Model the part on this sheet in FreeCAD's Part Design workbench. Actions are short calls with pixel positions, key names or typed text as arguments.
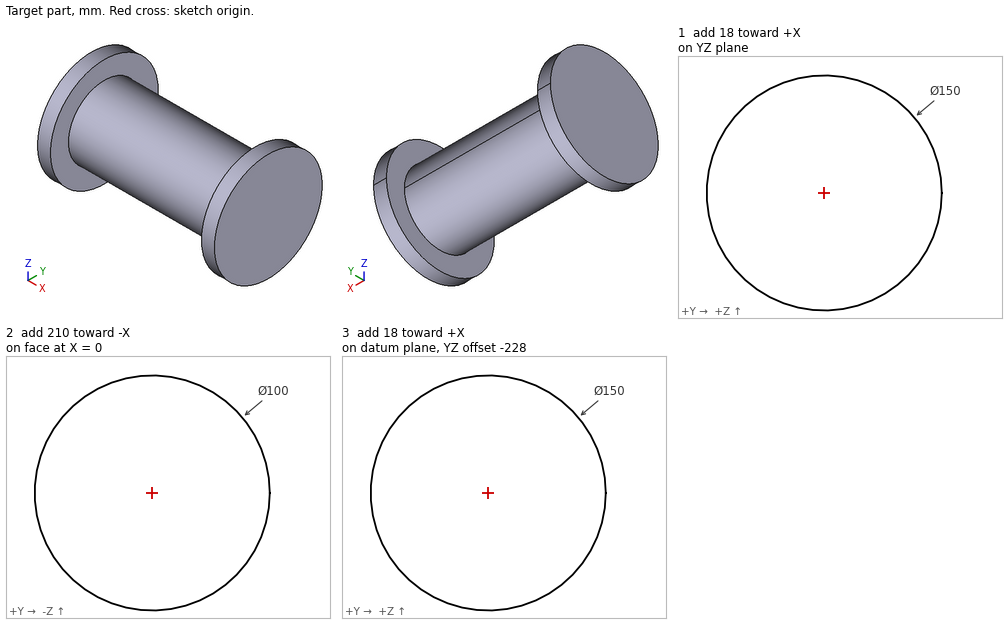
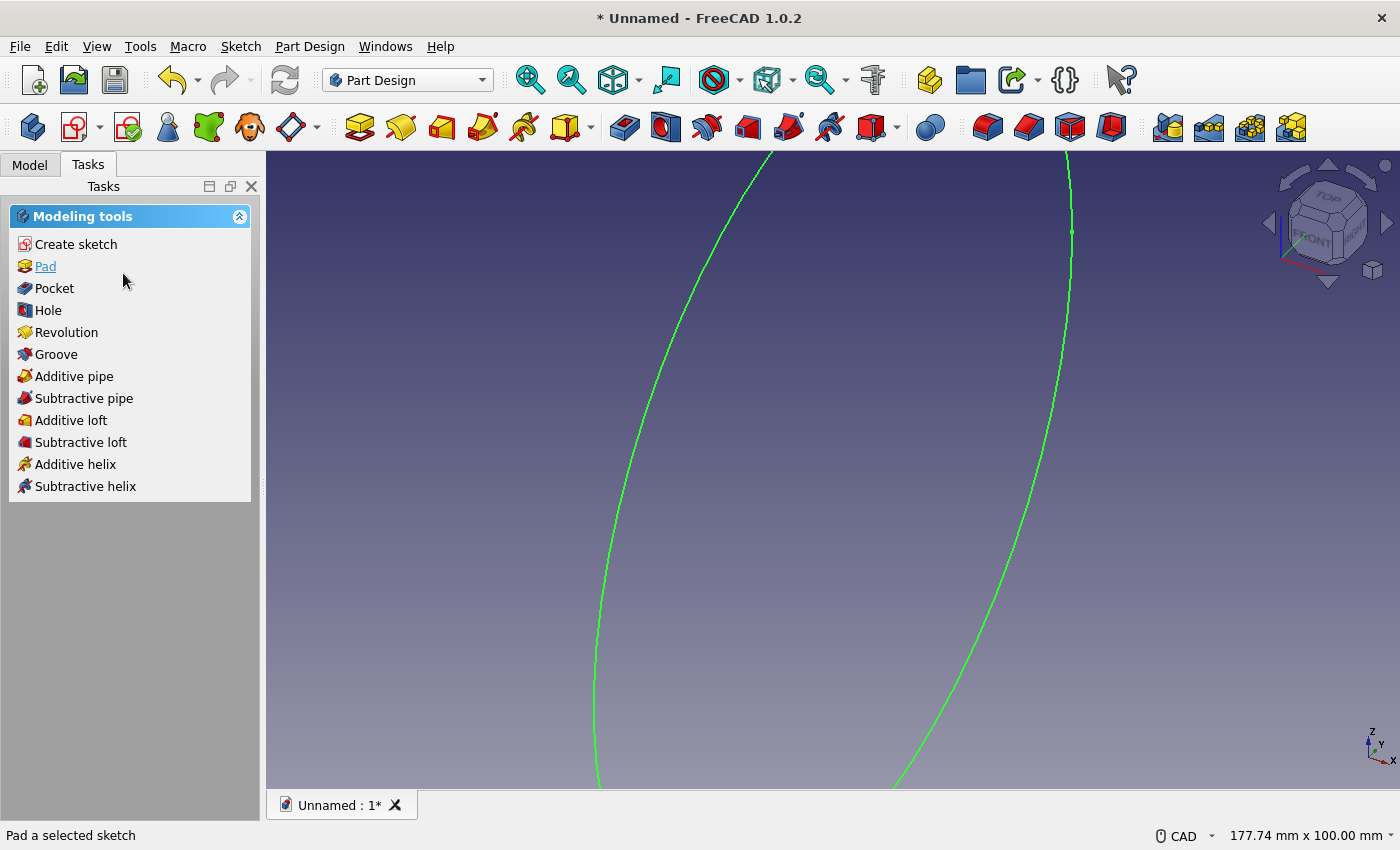
click(360, 128)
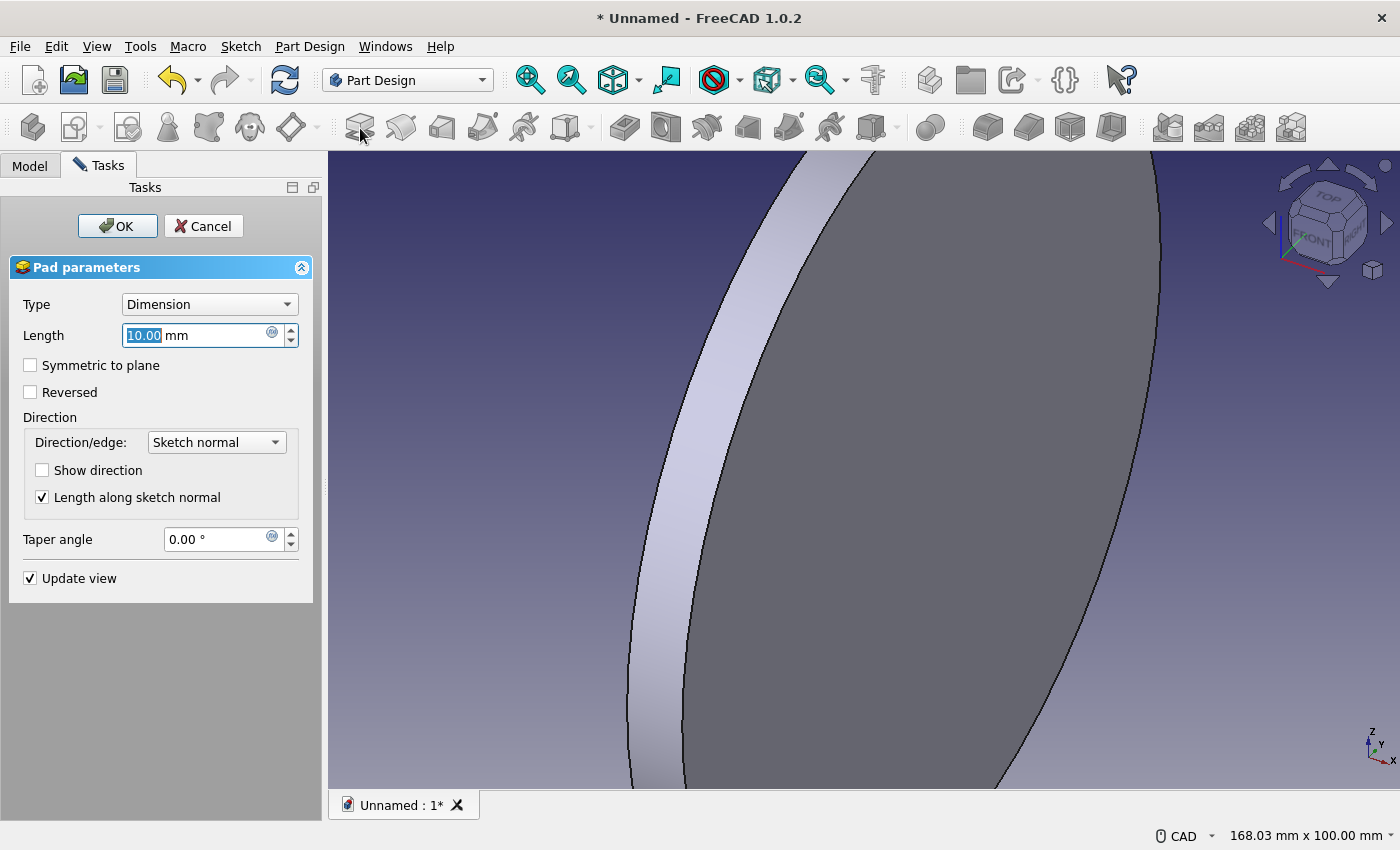
text(18)
key(Tab)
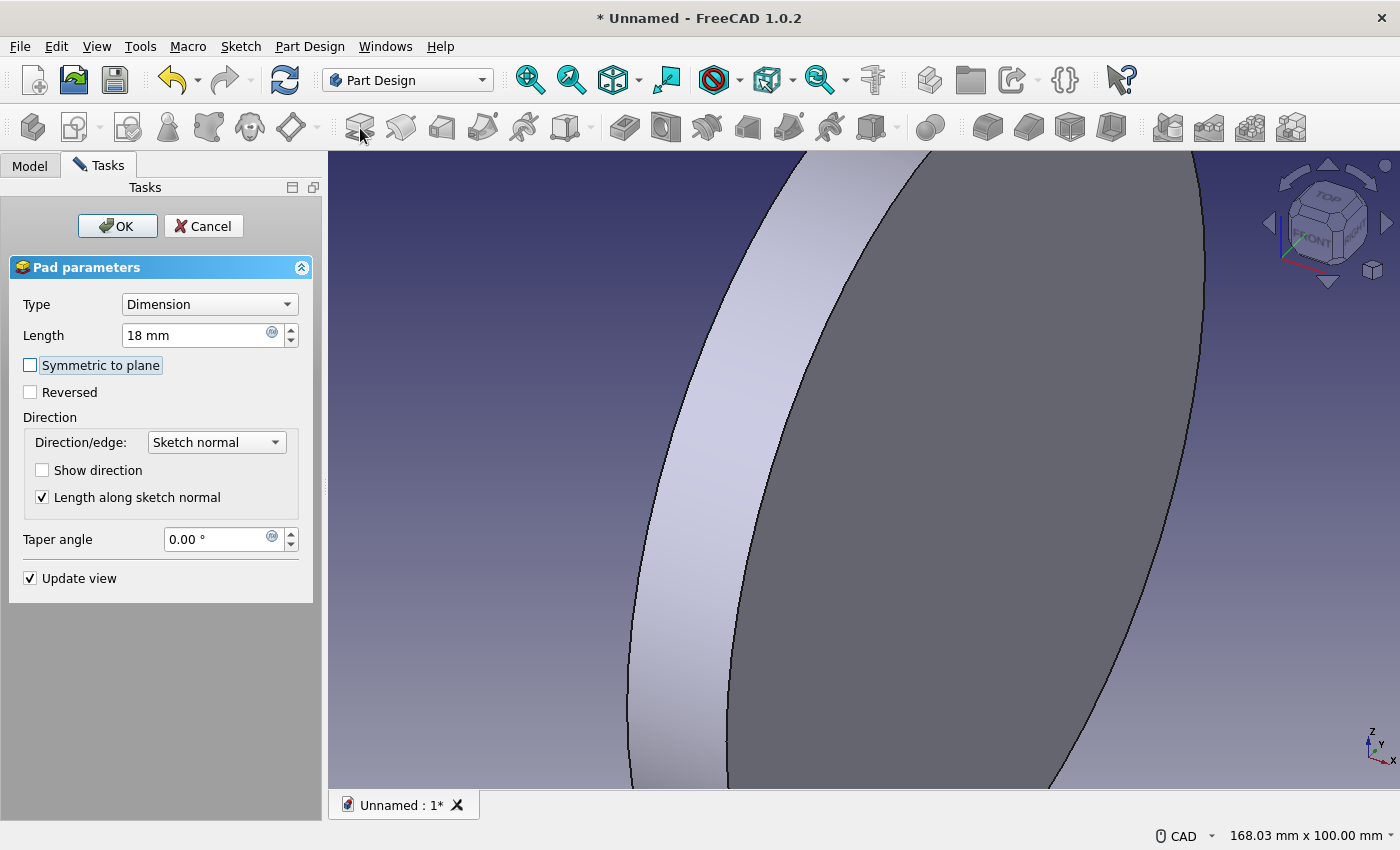
click(118, 226)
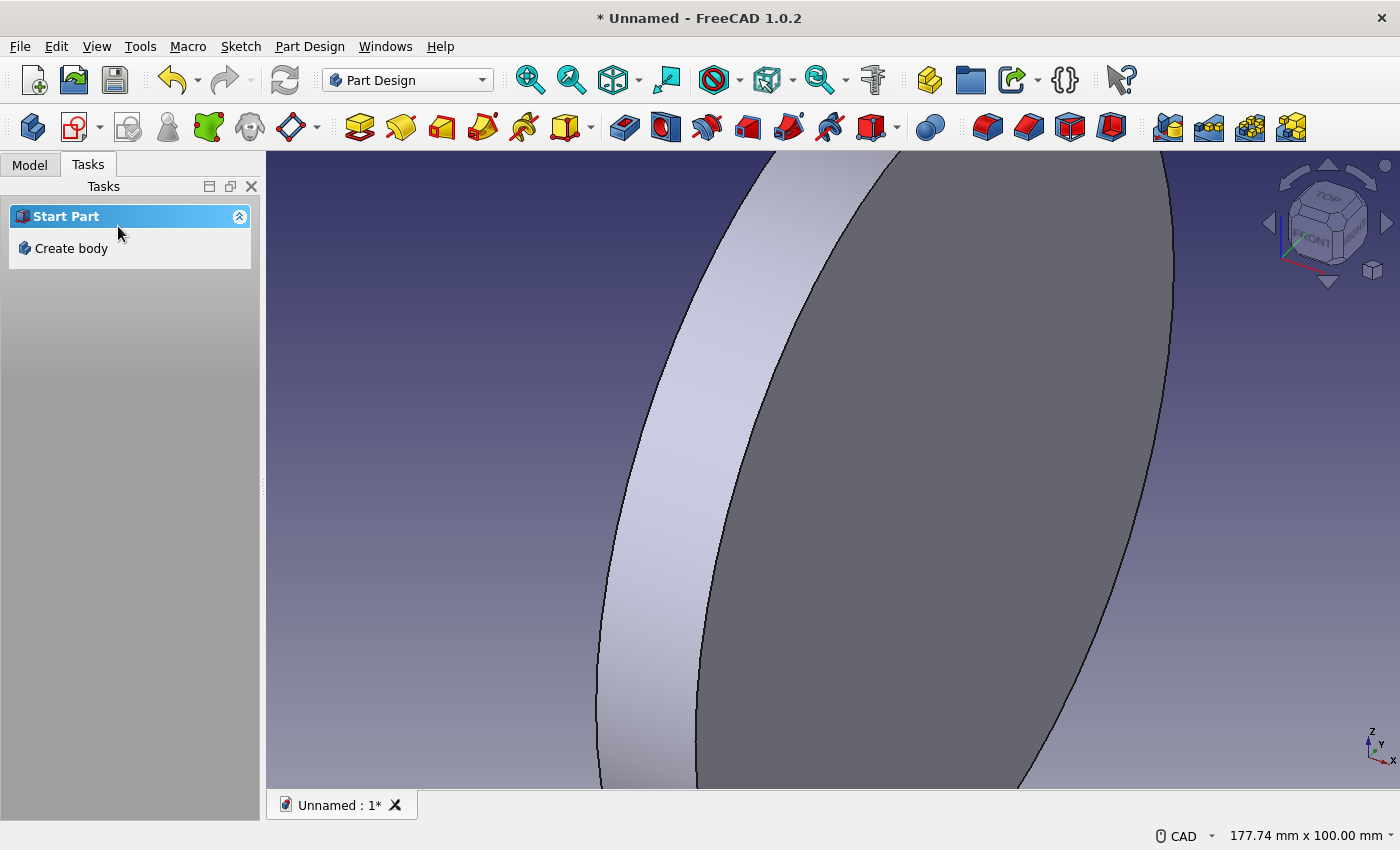
click(531, 80)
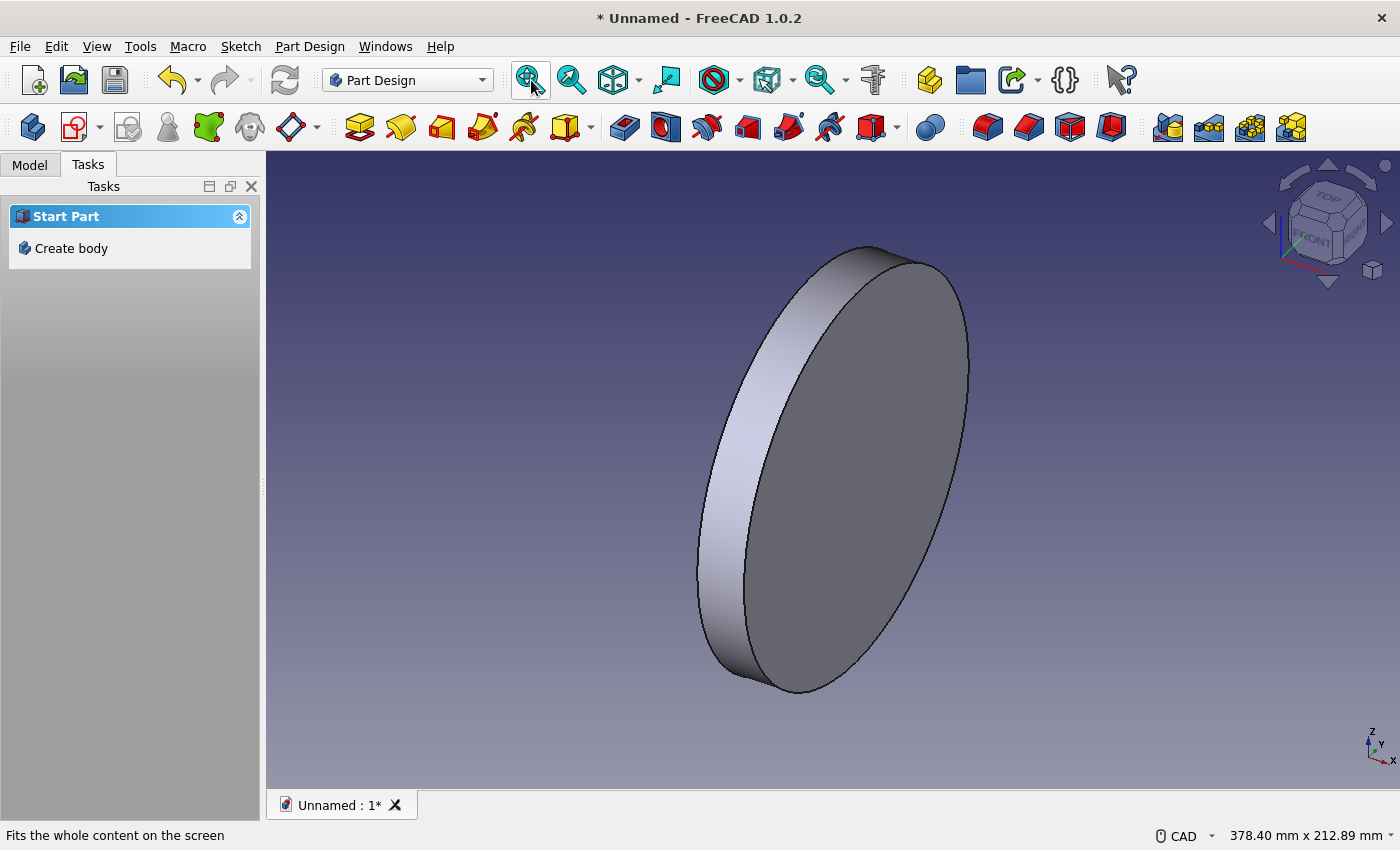
key(6)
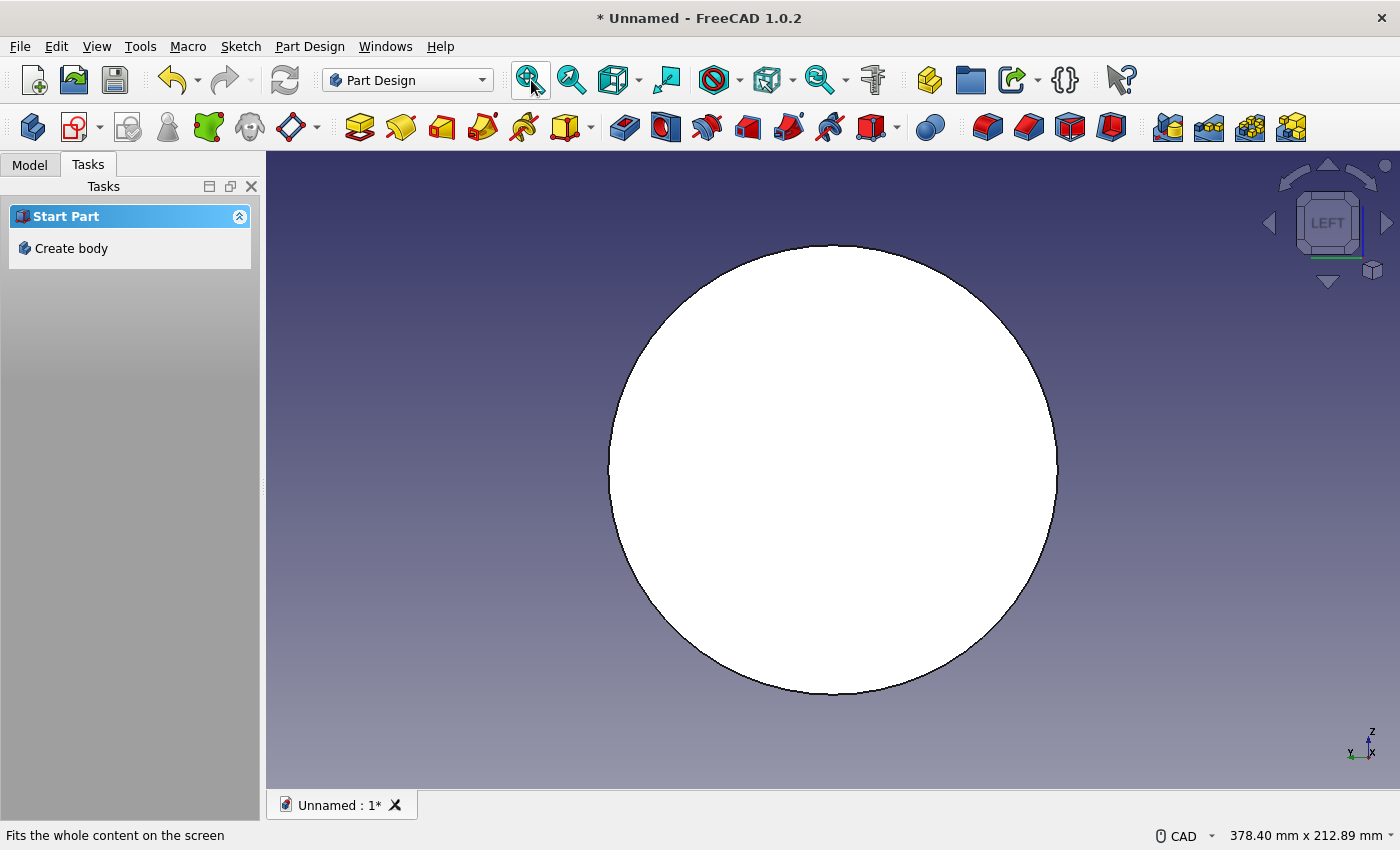
click(833, 469)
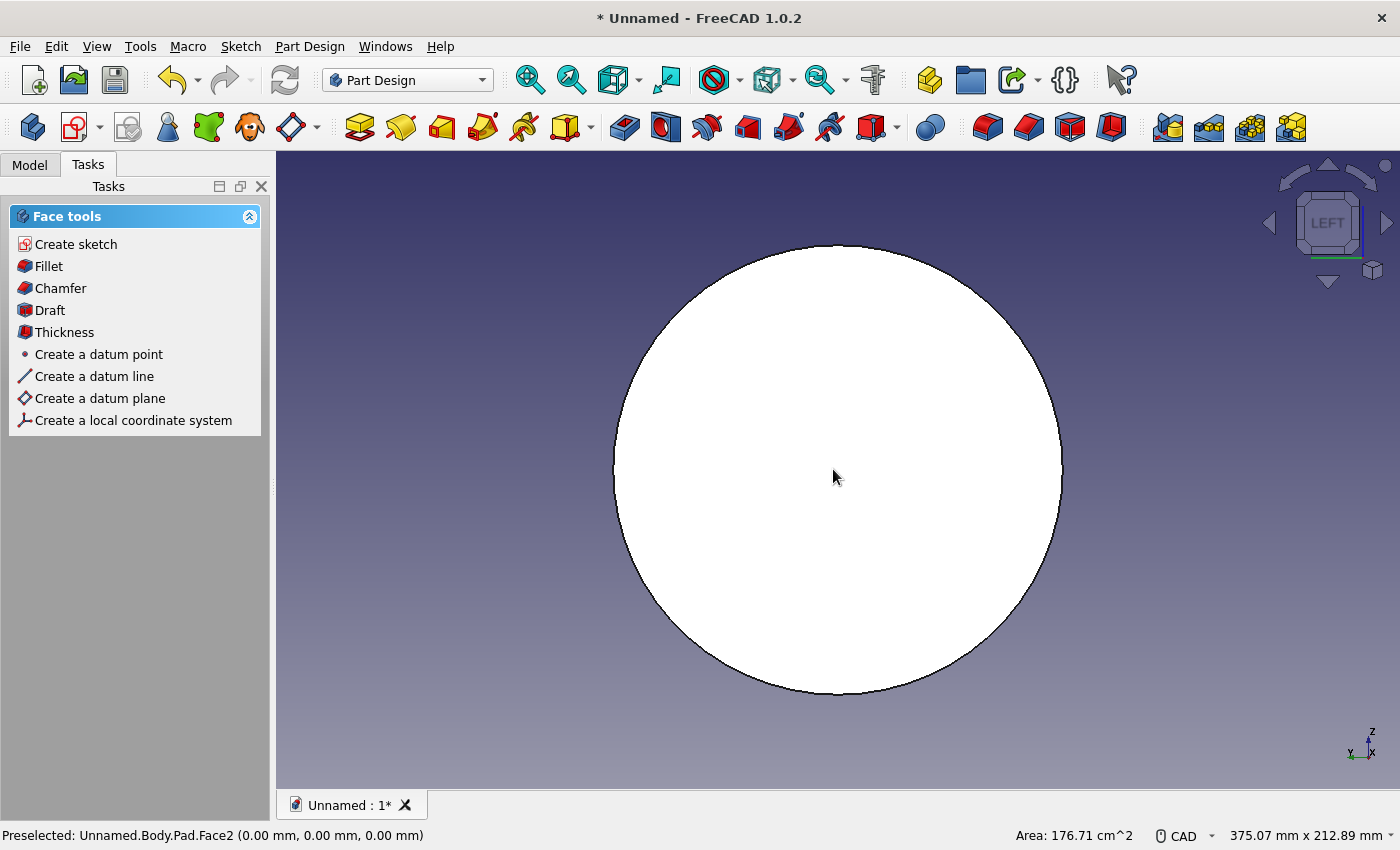
click(74, 128)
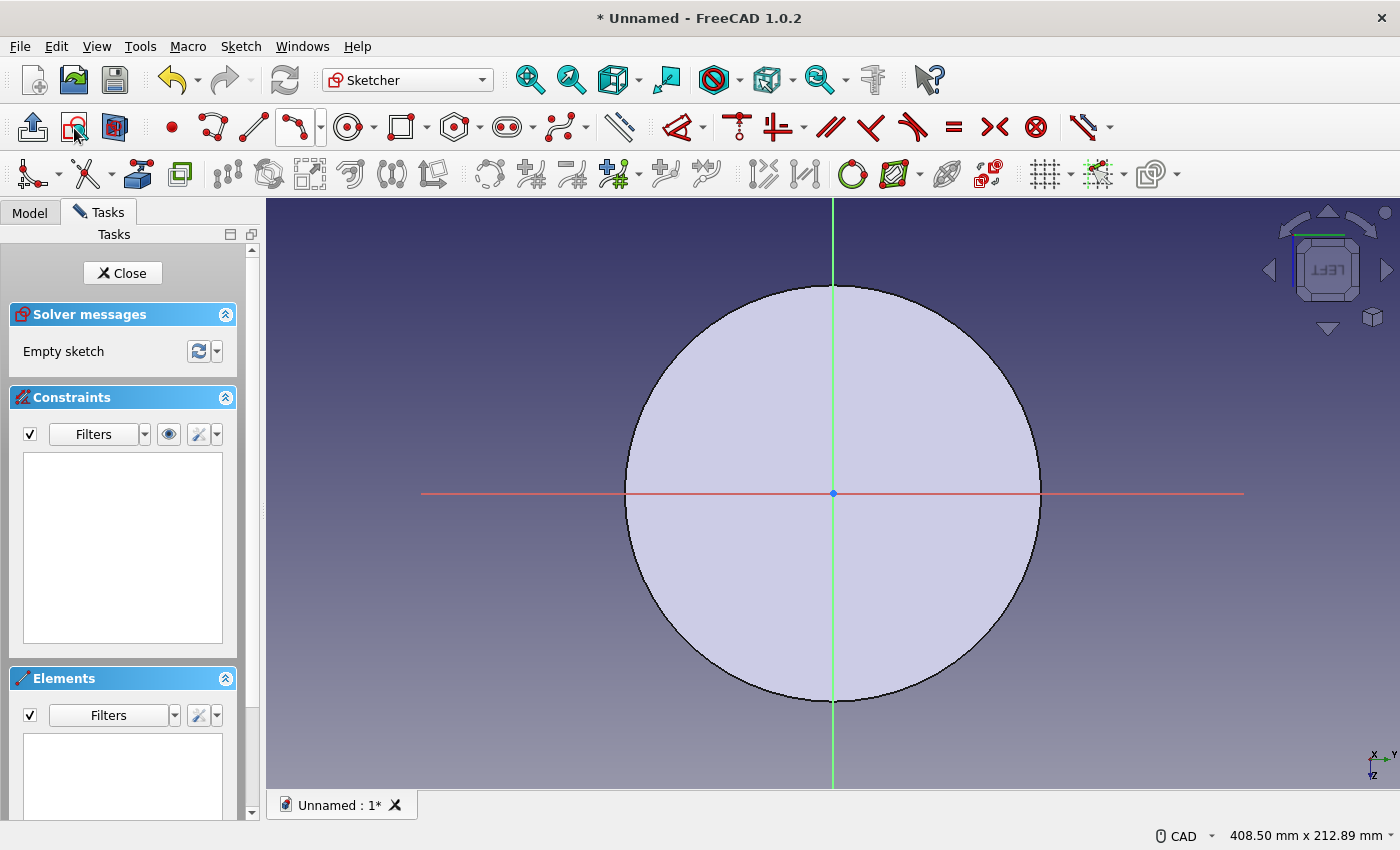
scroll(972, 493, up, 2)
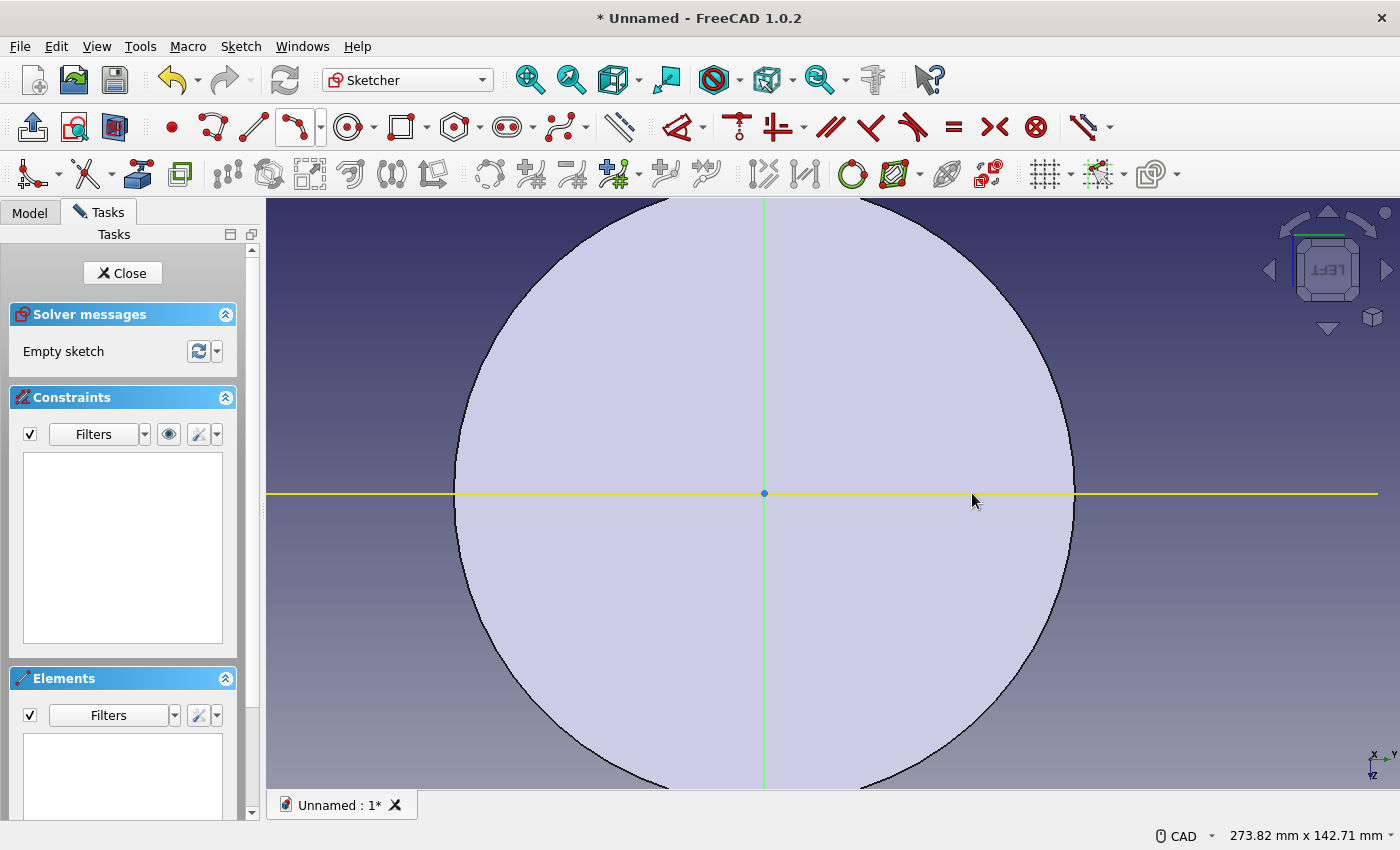
key(g)
key(c)